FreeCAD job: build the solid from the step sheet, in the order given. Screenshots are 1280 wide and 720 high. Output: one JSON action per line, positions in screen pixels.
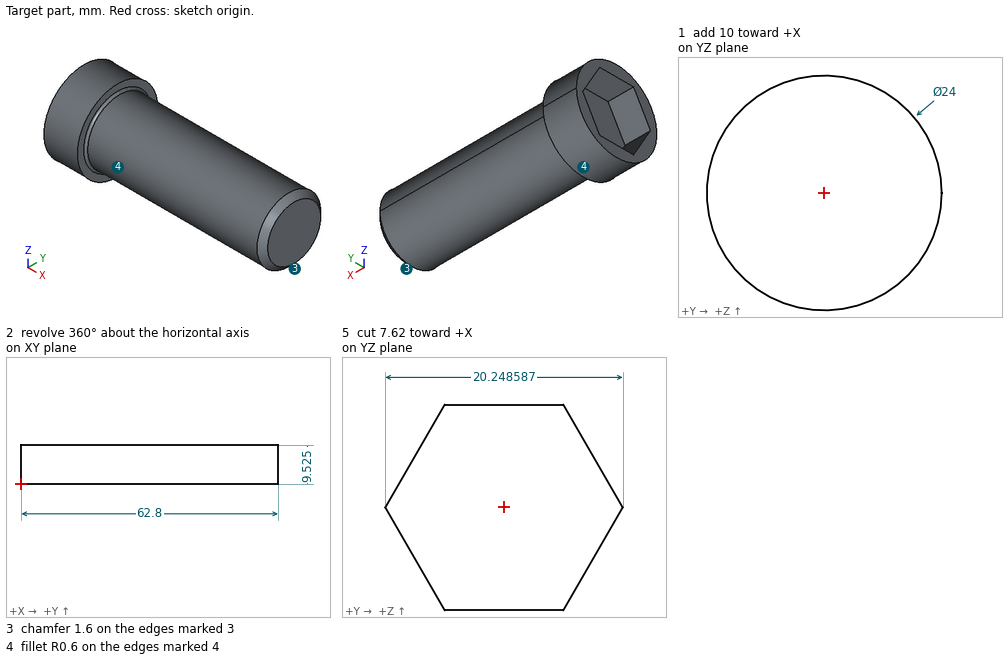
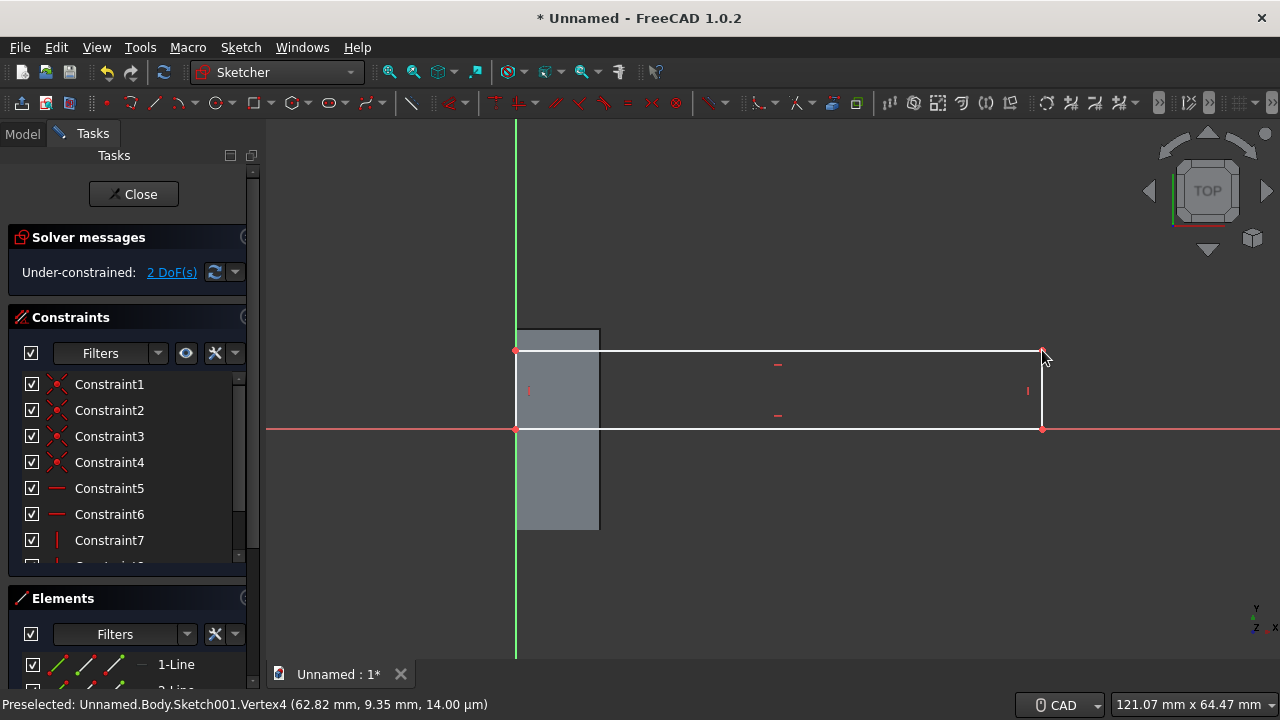
{"action": "left_click", "coordinate": [674, 429]}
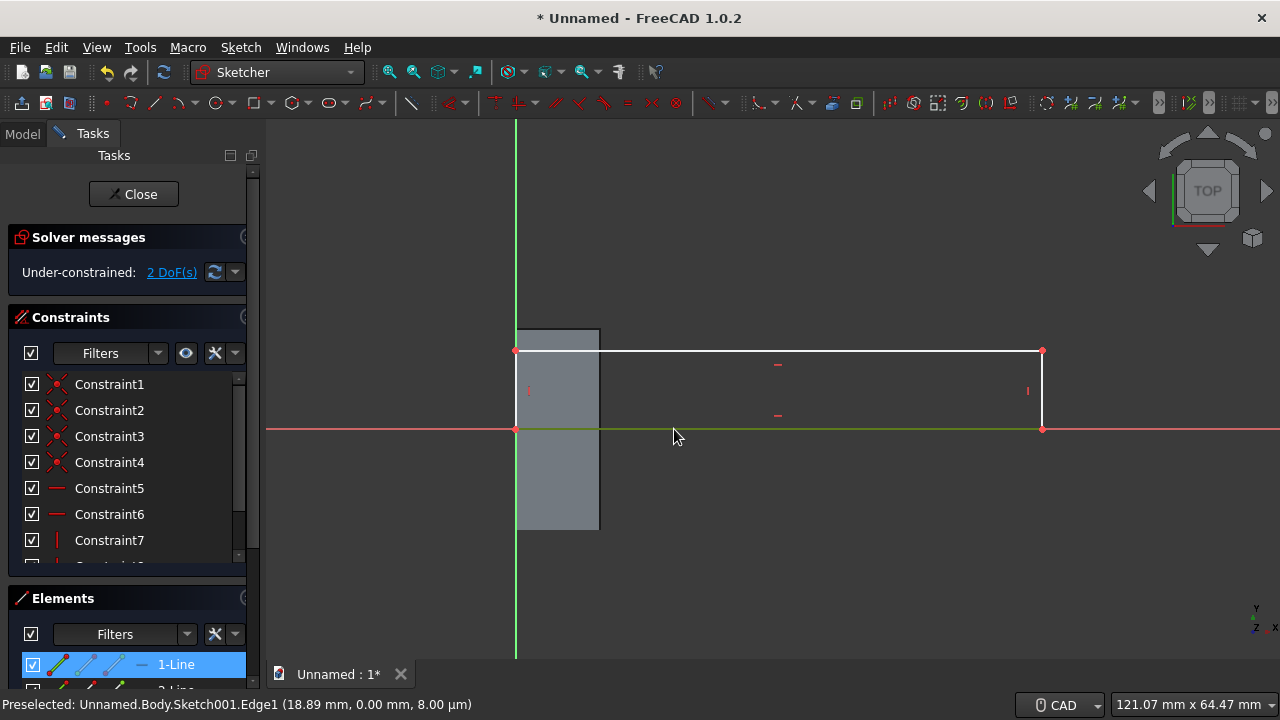
{"action": "key", "text": "l"}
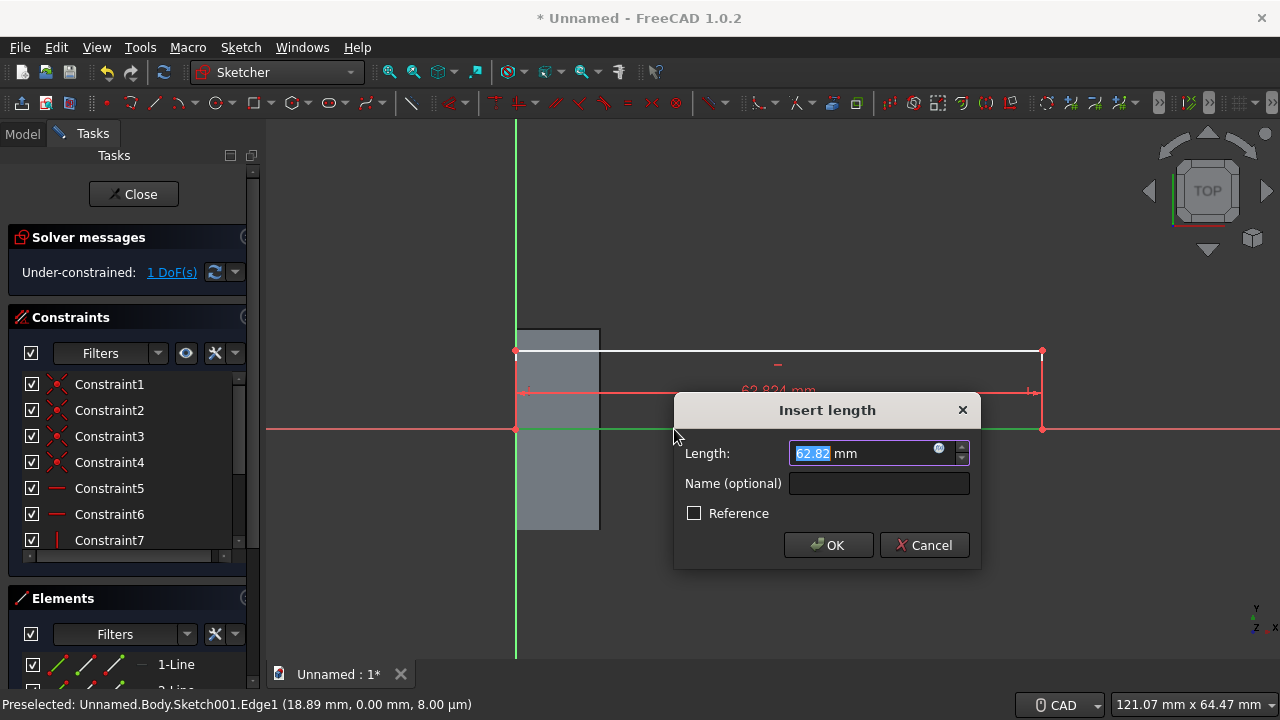
{"action": "type", "text": "62.8"}
{"action": "key", "text": "Return"}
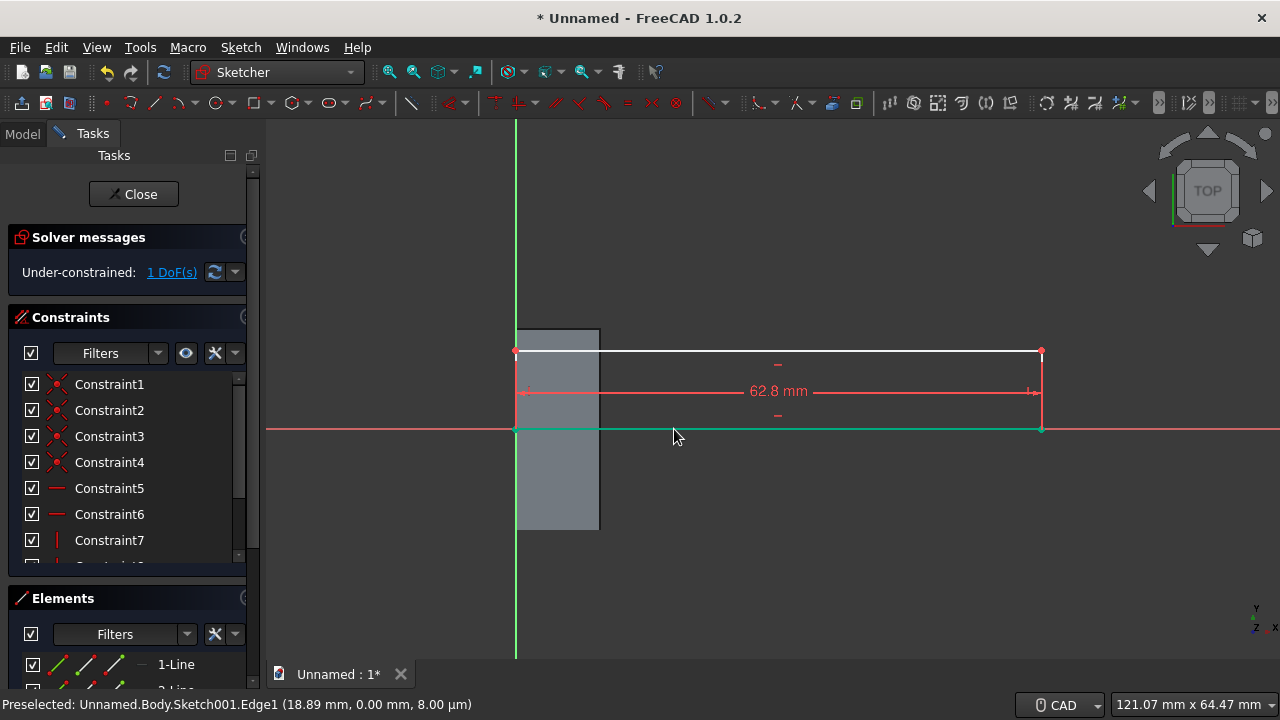
{"action": "left_click", "coordinate": [1042, 406]}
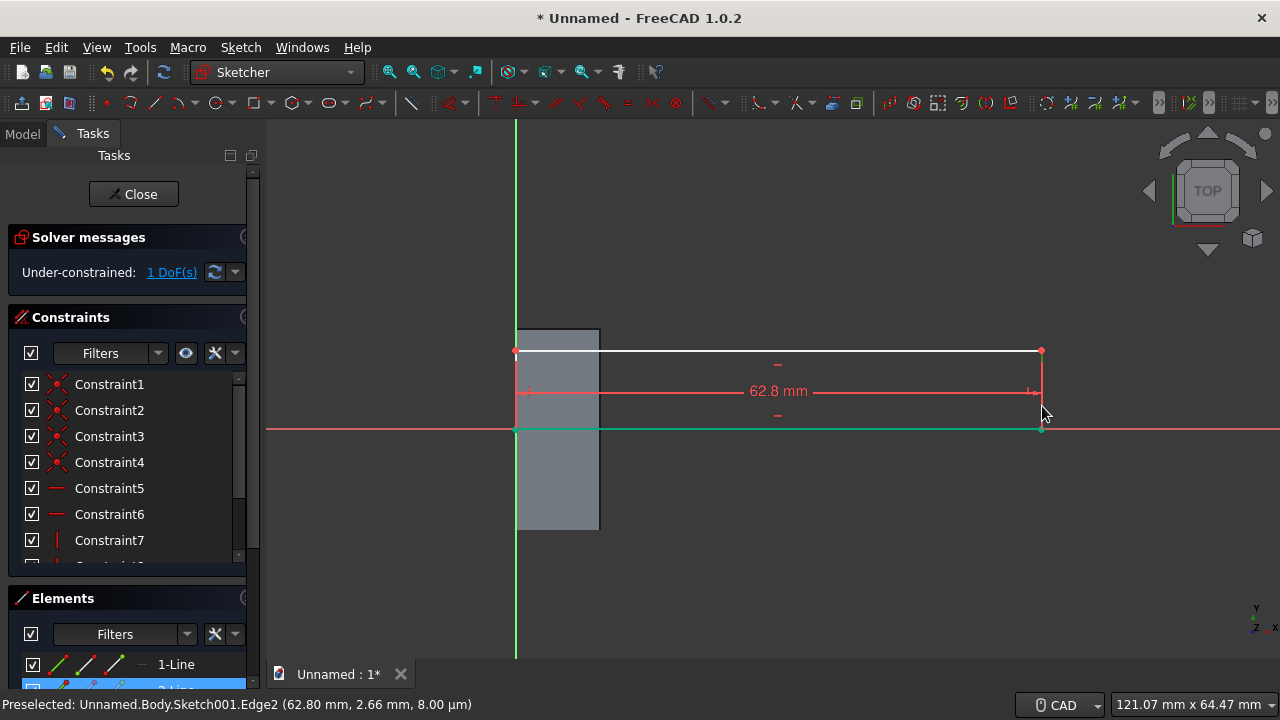
{"action": "key", "text": "i"}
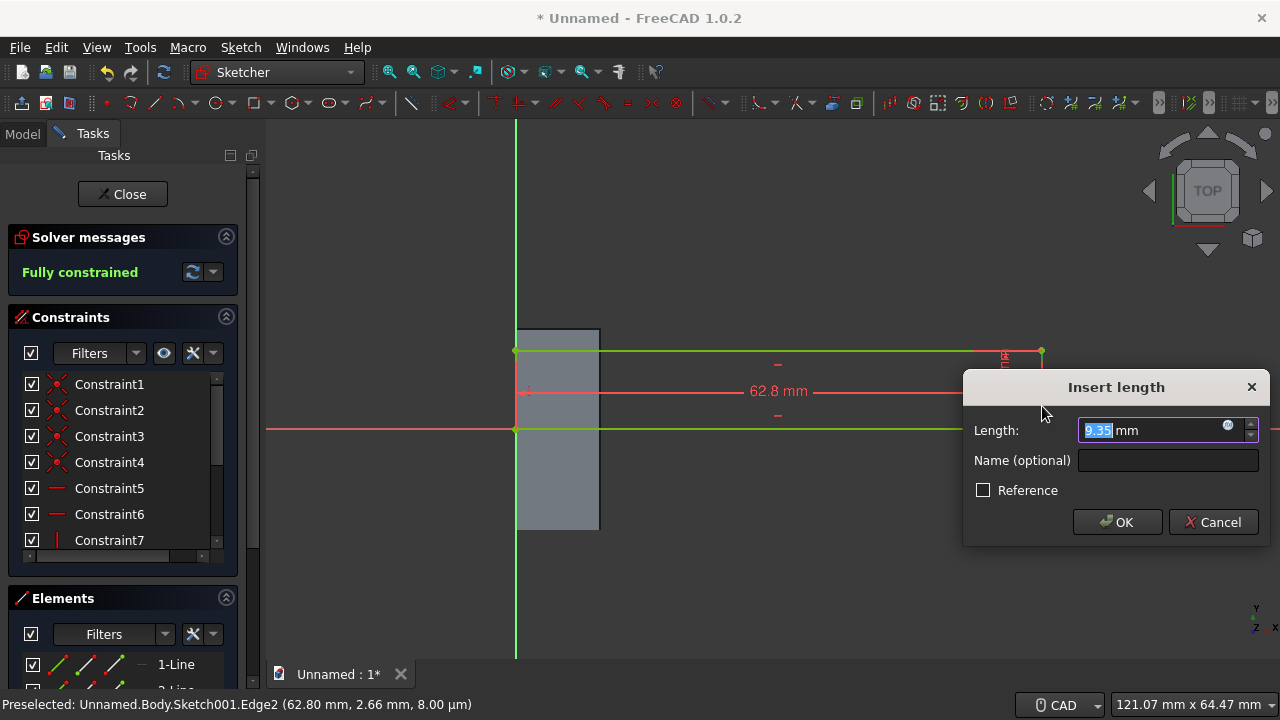
{"action": "type", "text": "9.525"}
{"action": "key", "text": "Return"}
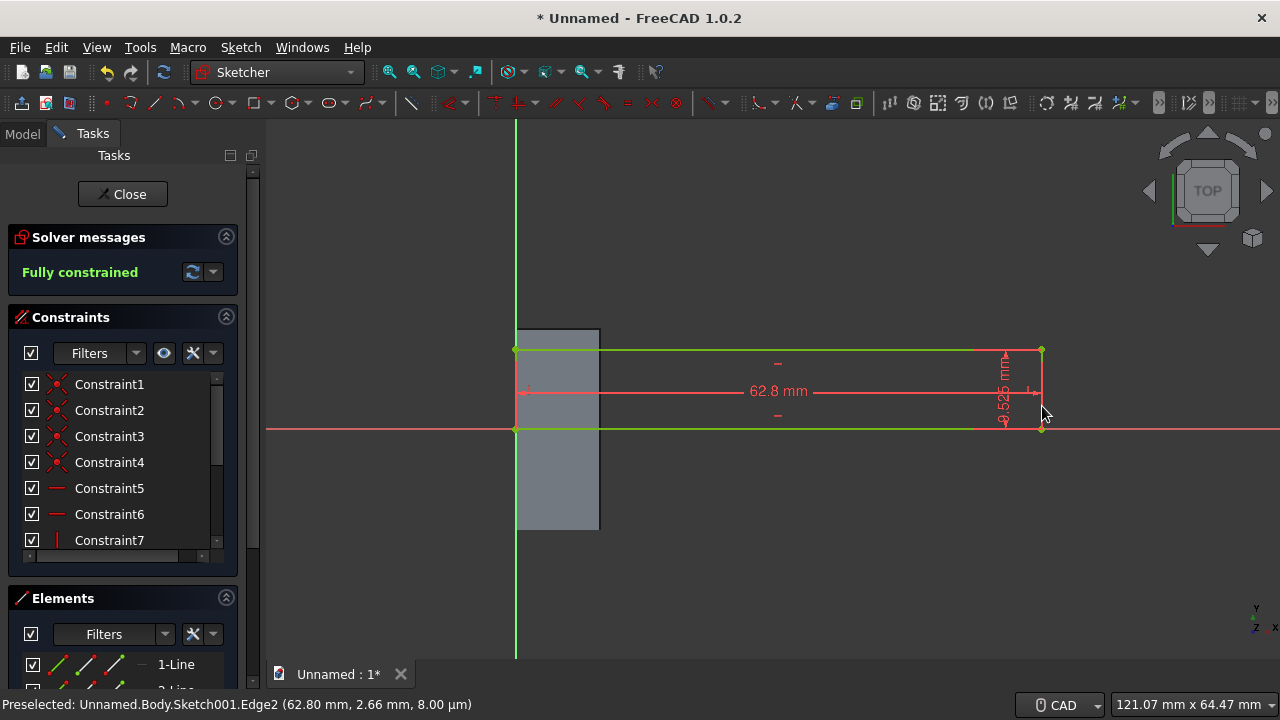
{"action": "left_click", "coordinate": [123, 194]}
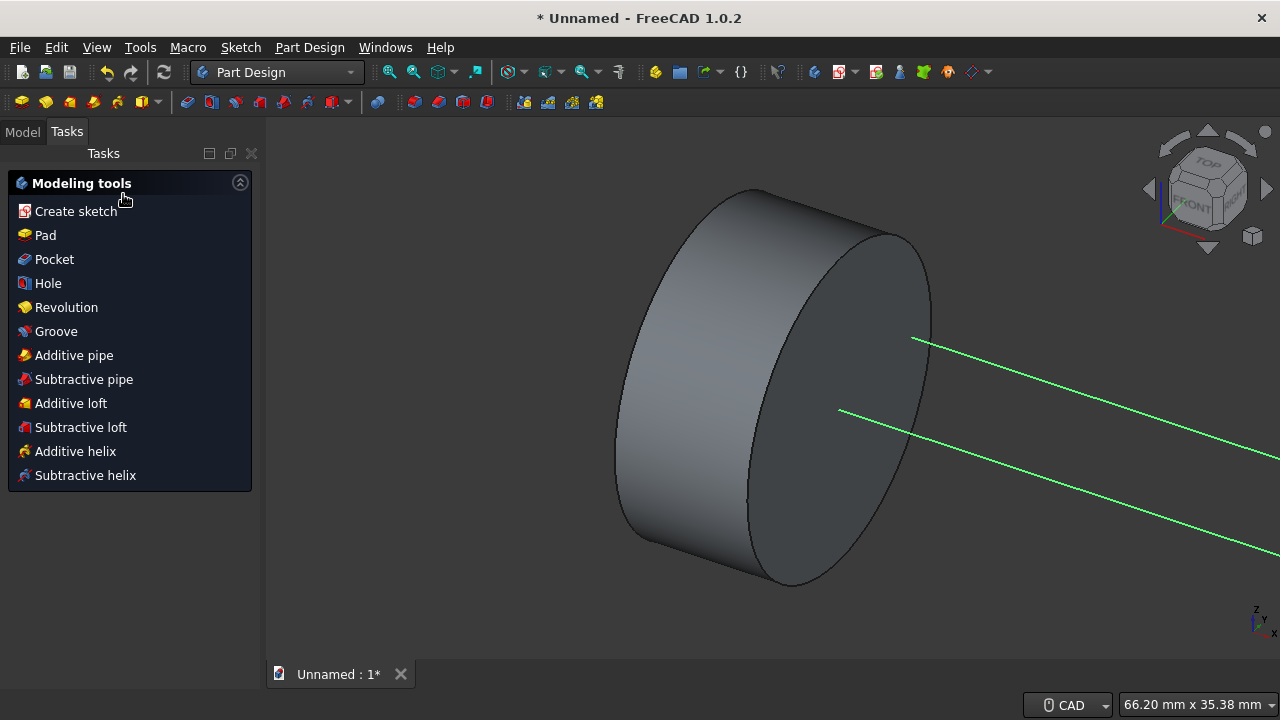
{"action": "left_click", "coordinate": [46, 102]}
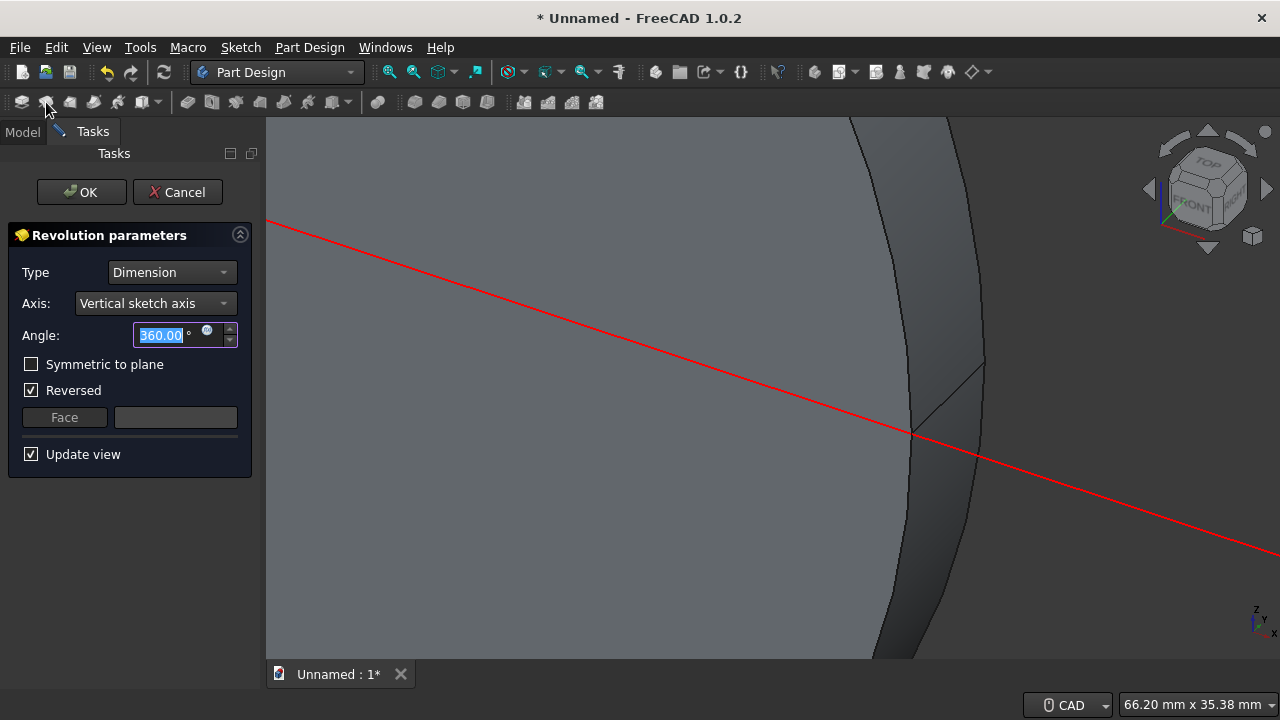
{"action": "left_click", "coordinate": [156, 304]}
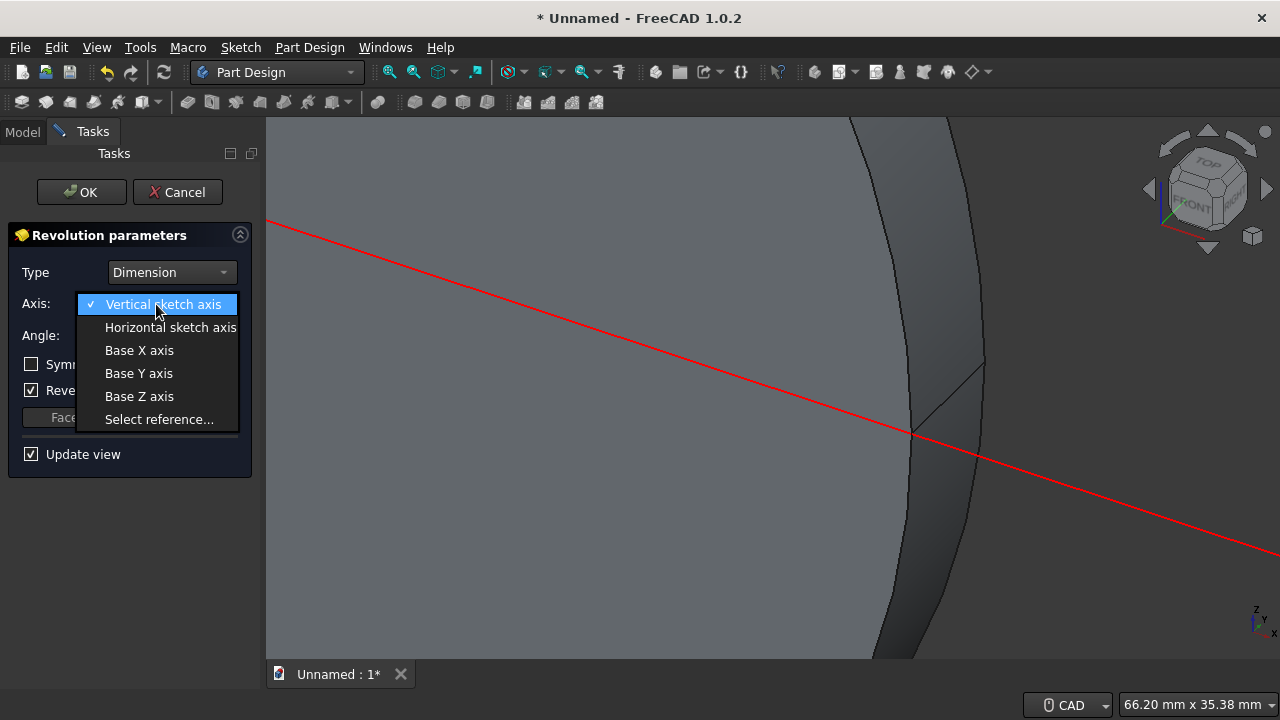
{"action": "left_click", "coordinate": [156, 328]}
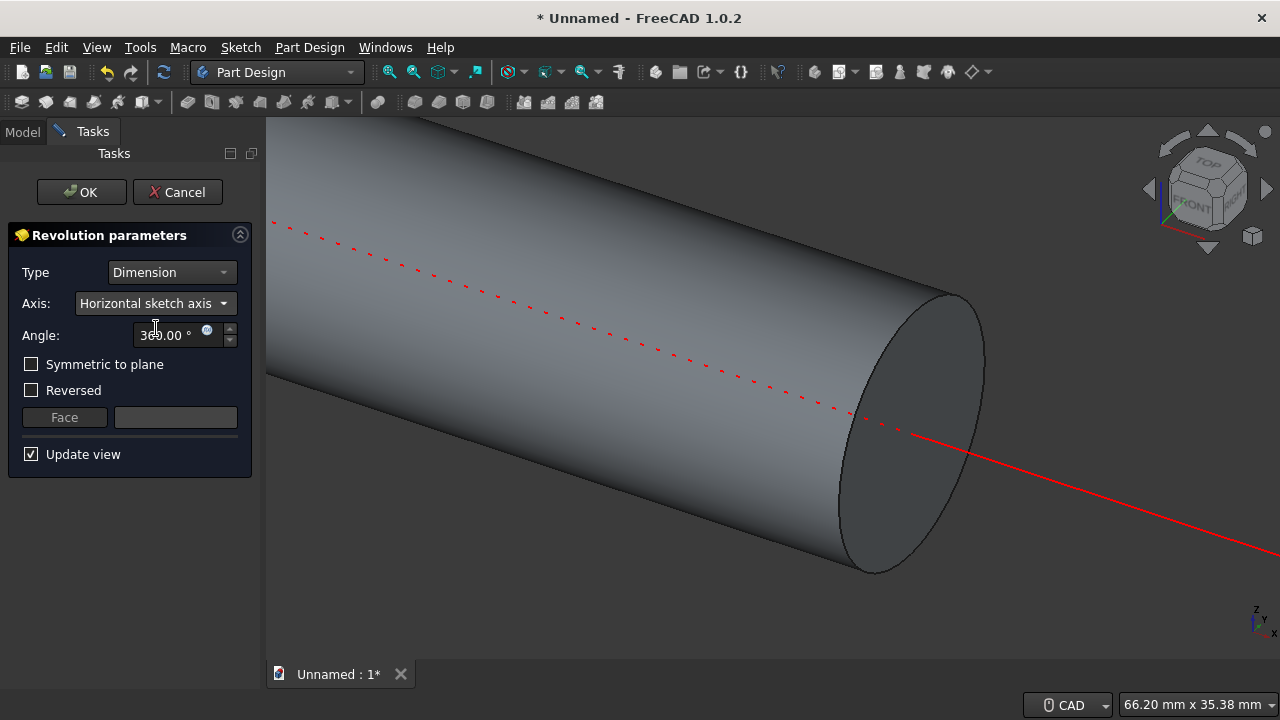
{"action": "left_click", "coordinate": [82, 192]}